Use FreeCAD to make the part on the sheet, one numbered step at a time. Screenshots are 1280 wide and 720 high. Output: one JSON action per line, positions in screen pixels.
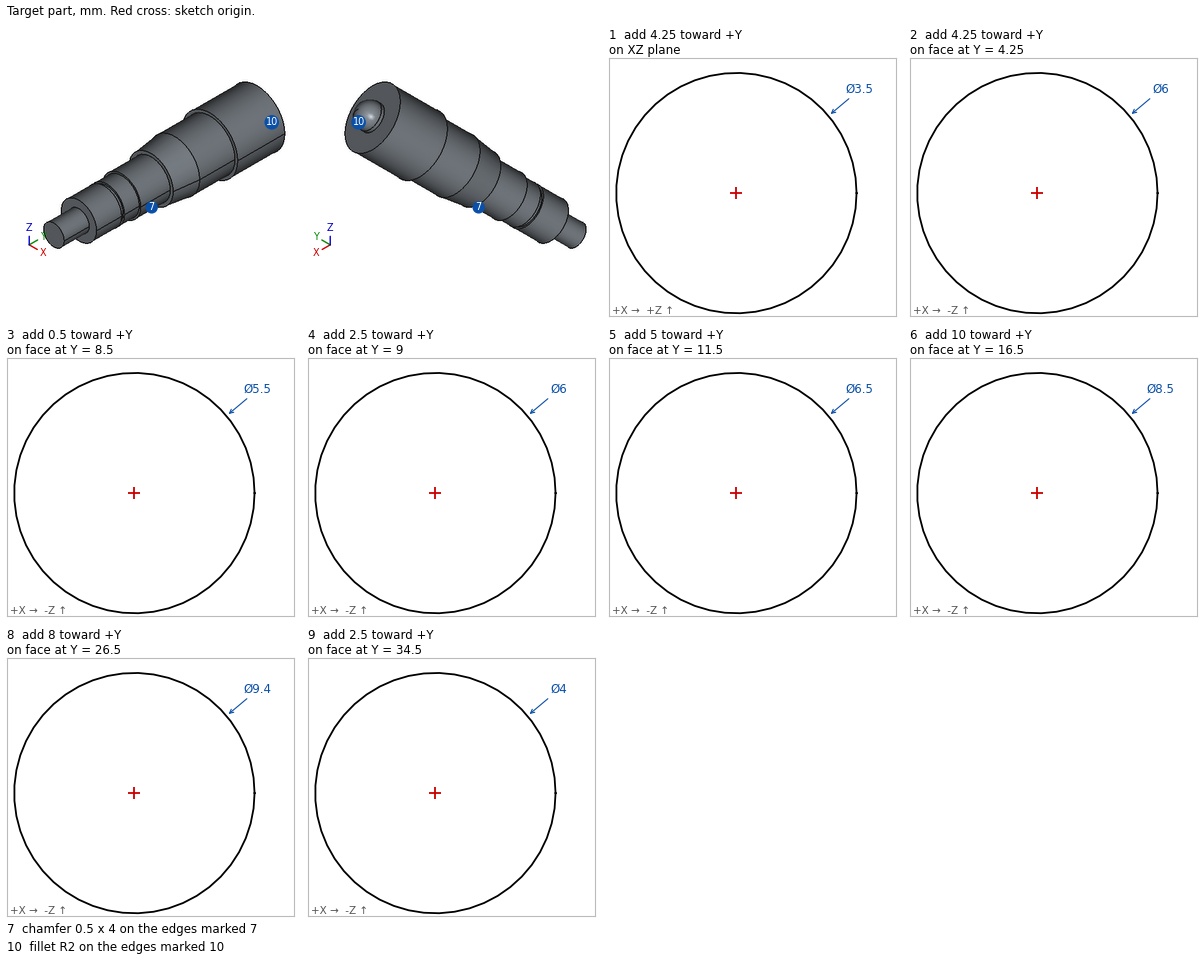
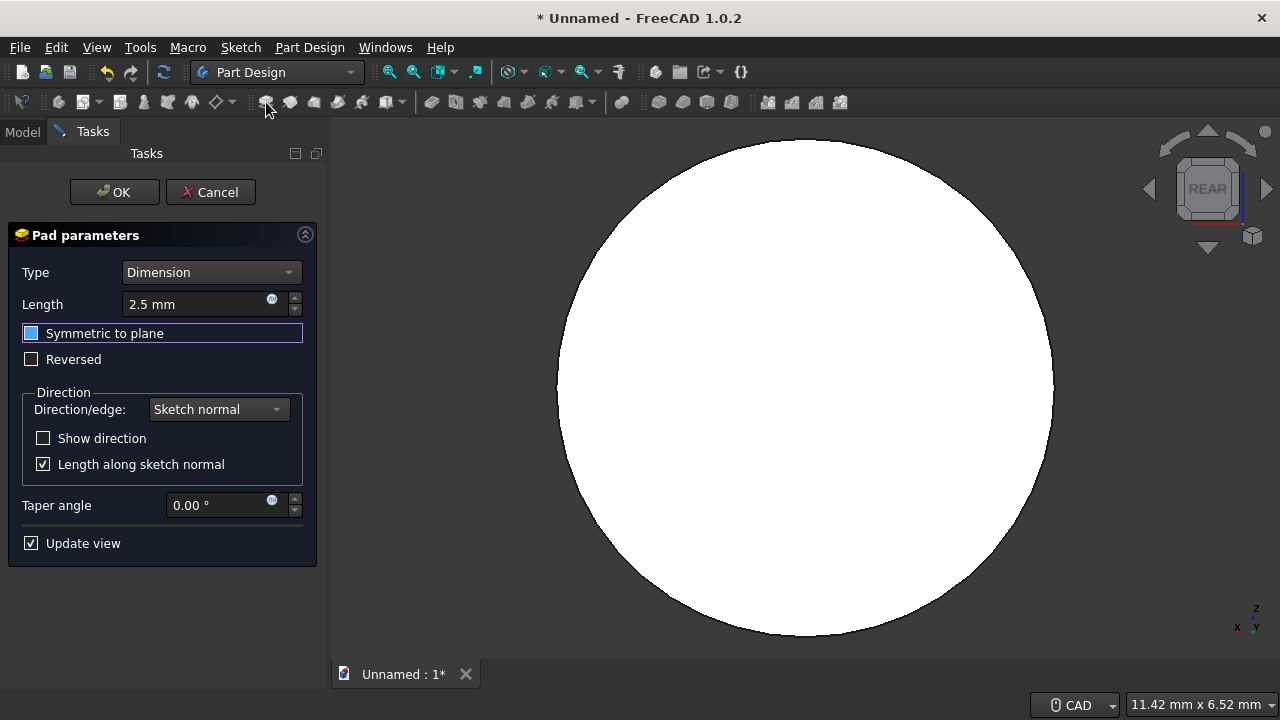
{"action": "left_click", "coordinate": [115, 192]}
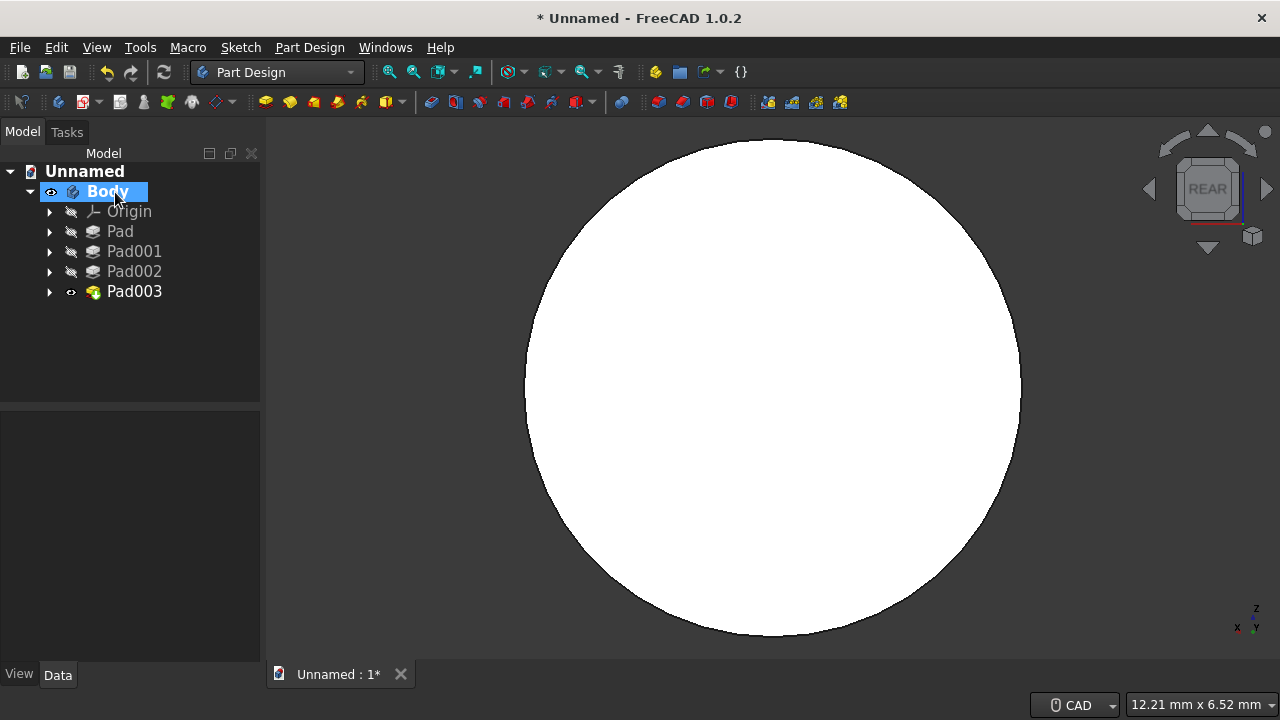
{"action": "left_click", "coordinate": [773, 387]}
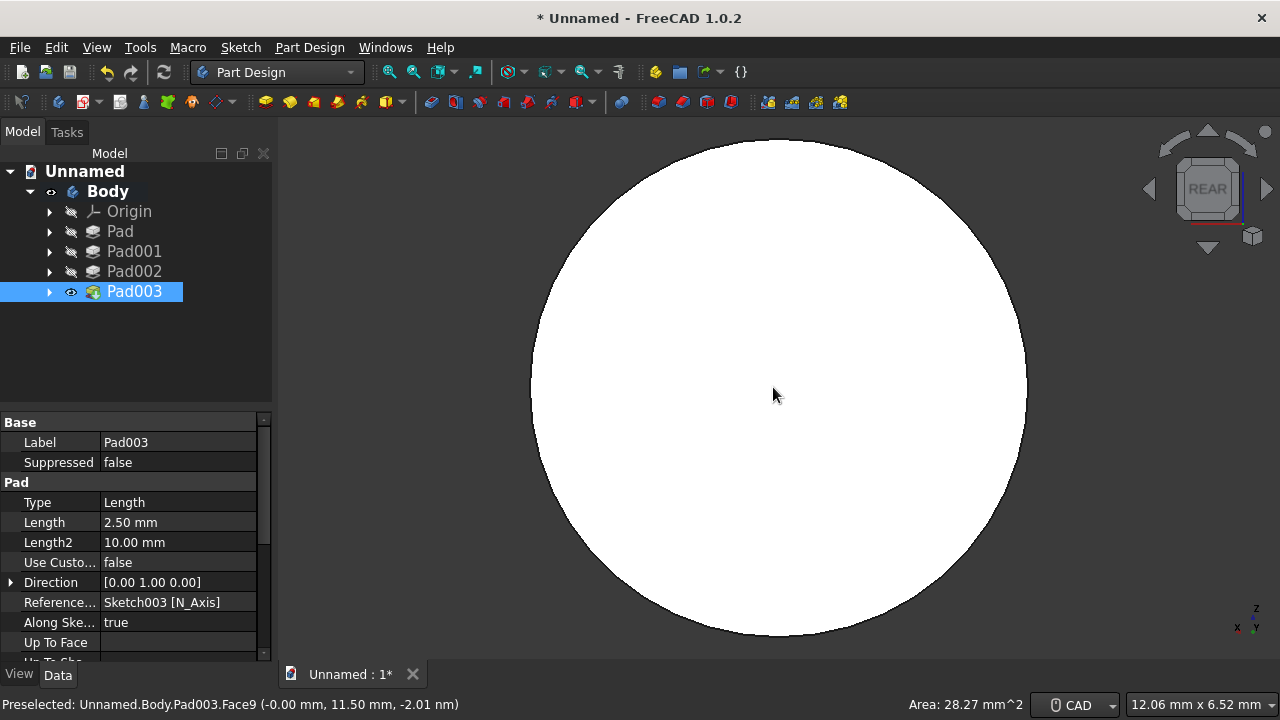
{"action": "left_click", "coordinate": [84, 102]}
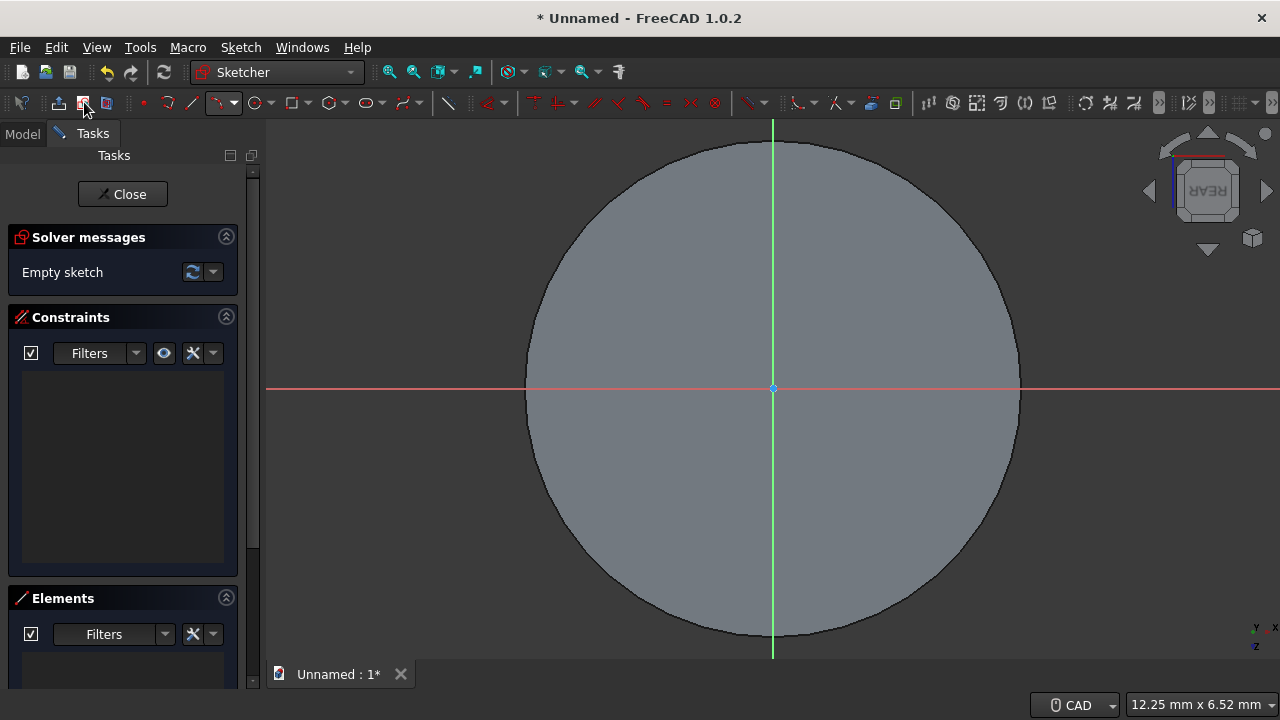
{"action": "scroll", "coordinate": [565, 389], "scroll_direction": "down", "scroll_amount": 2}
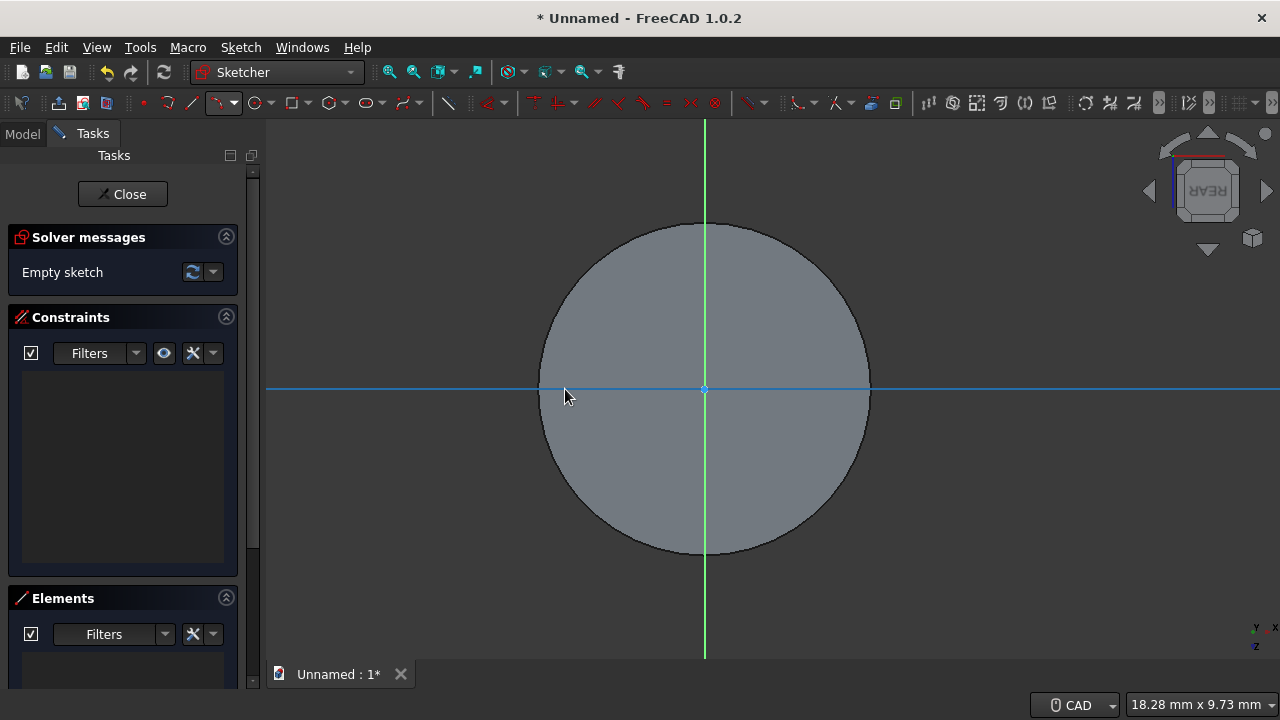
{"action": "left_click", "coordinate": [256, 104]}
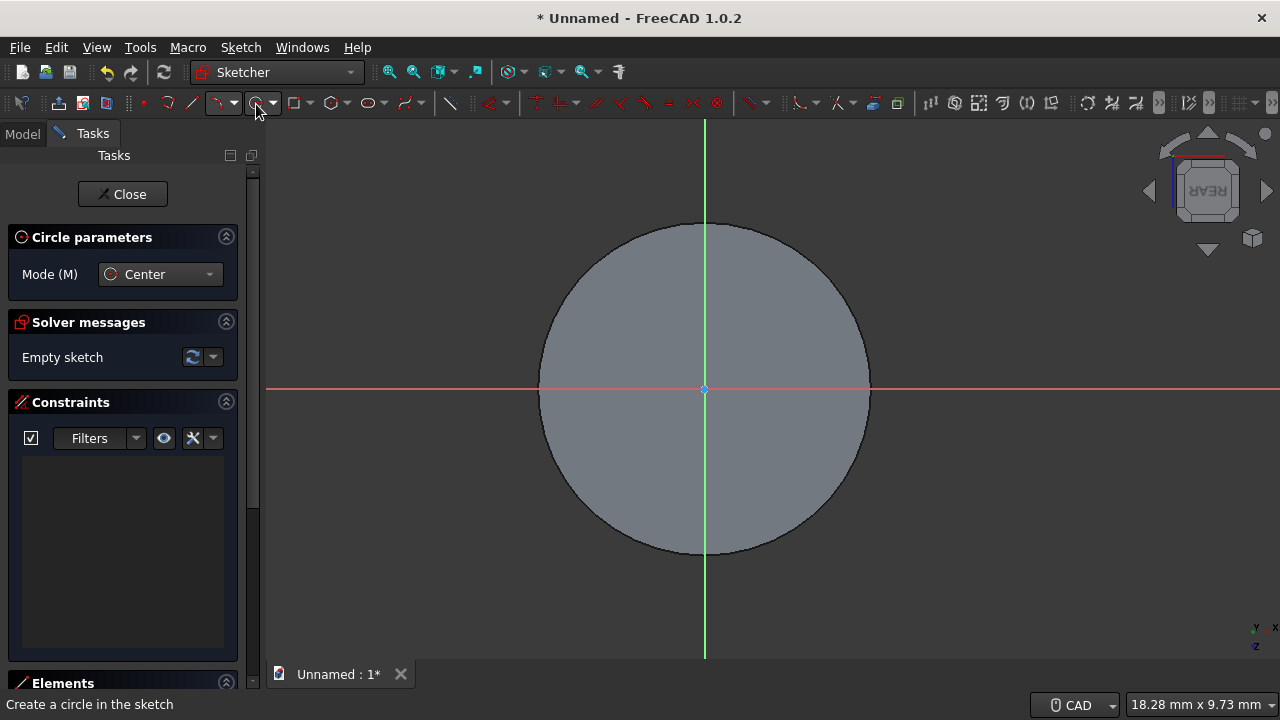
{"action": "left_click", "coordinate": [705, 389]}
{"action": "mouse_move", "coordinate": [832, 262]}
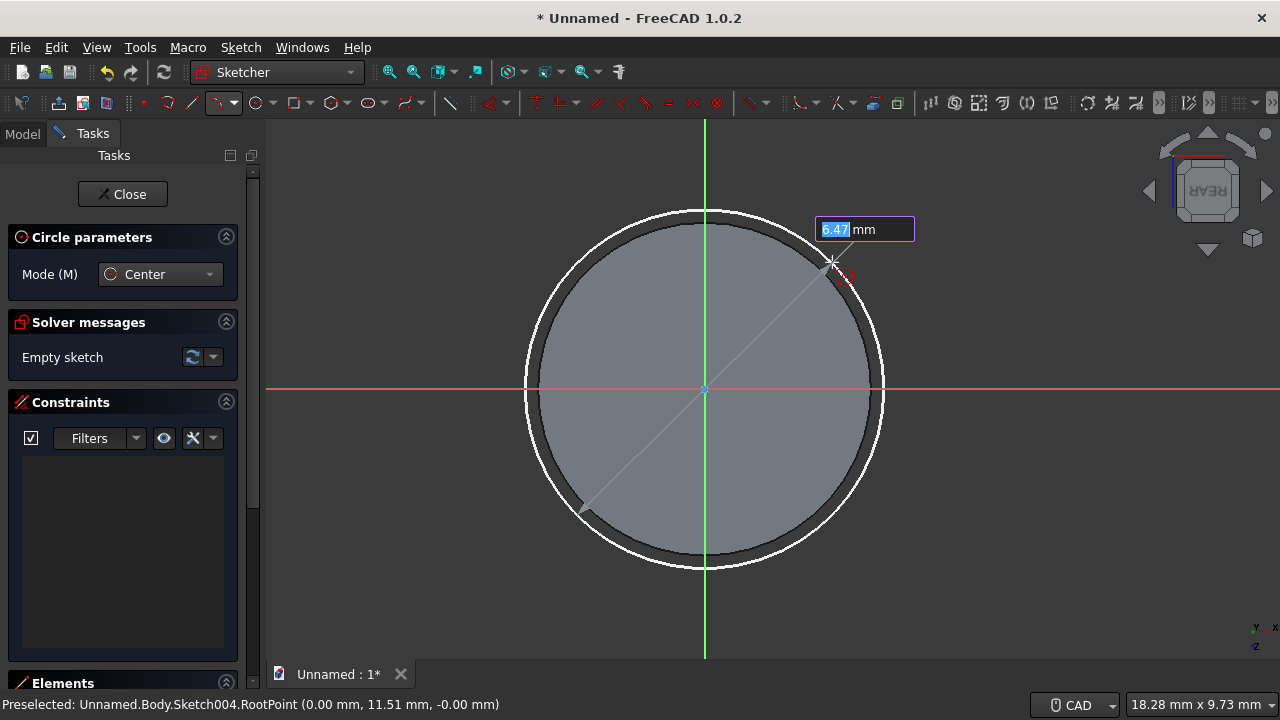
{"action": "type", "text": "6.5"}
{"action": "key", "text": "Return"}
{"action": "key", "text": "Escape"}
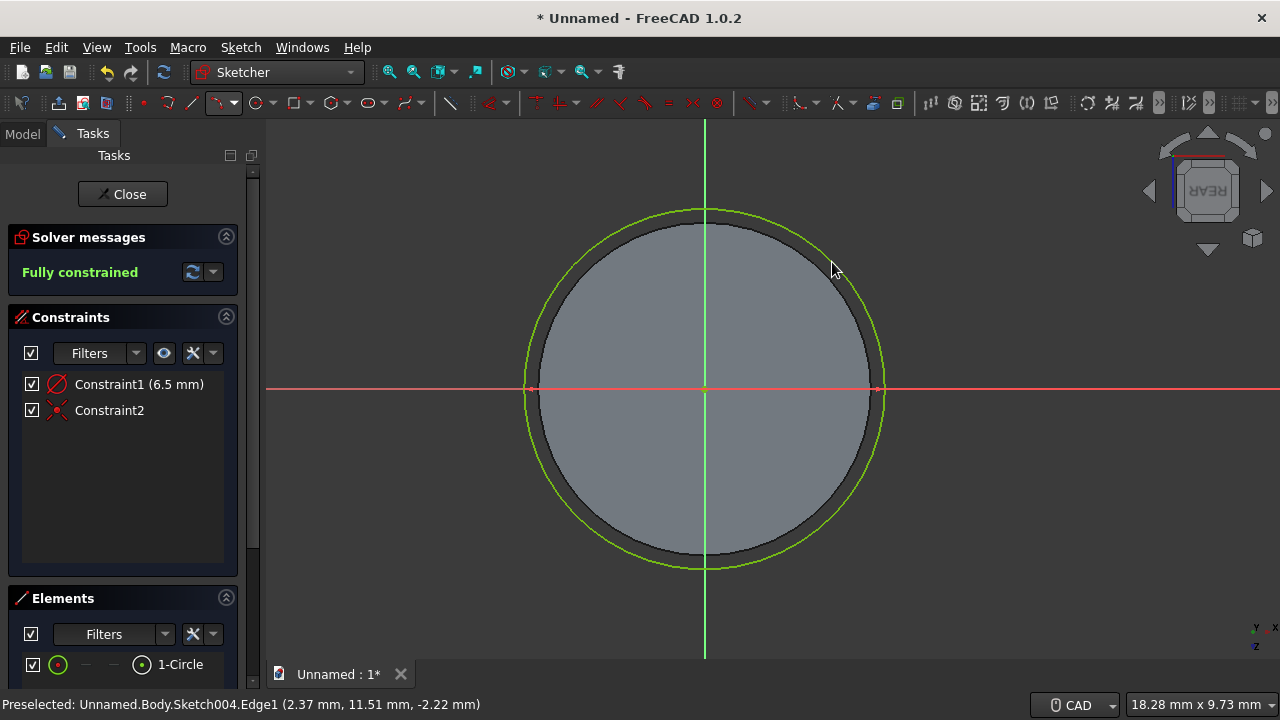
{"action": "left_click", "coordinate": [123, 194]}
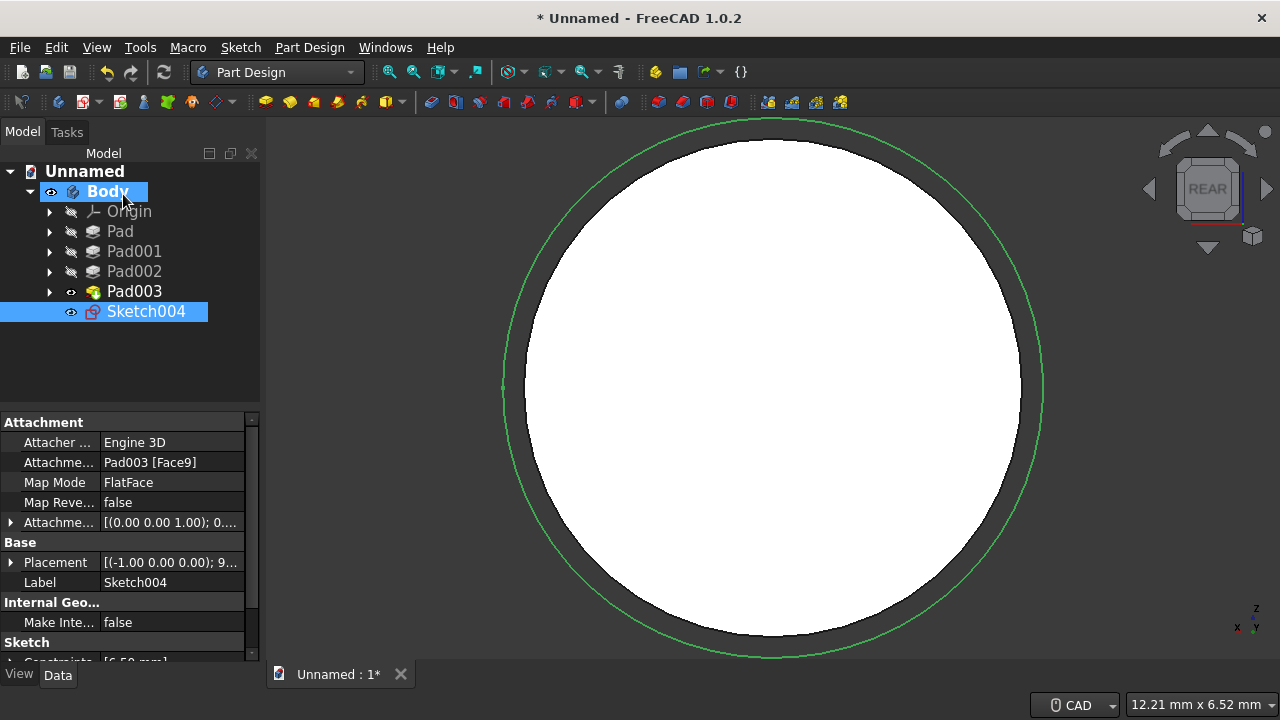
{"action": "left_click", "coordinate": [266, 102]}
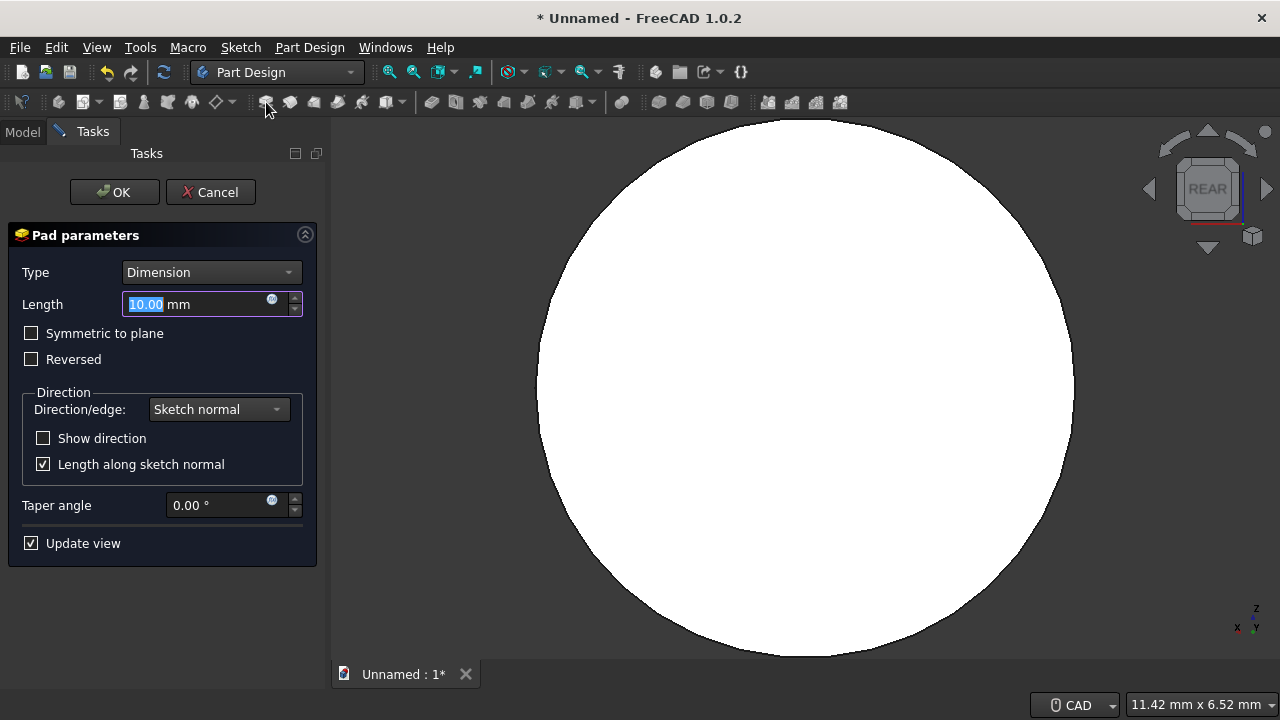
{"action": "type", "text": "5"}
{"action": "key", "text": "Tab"}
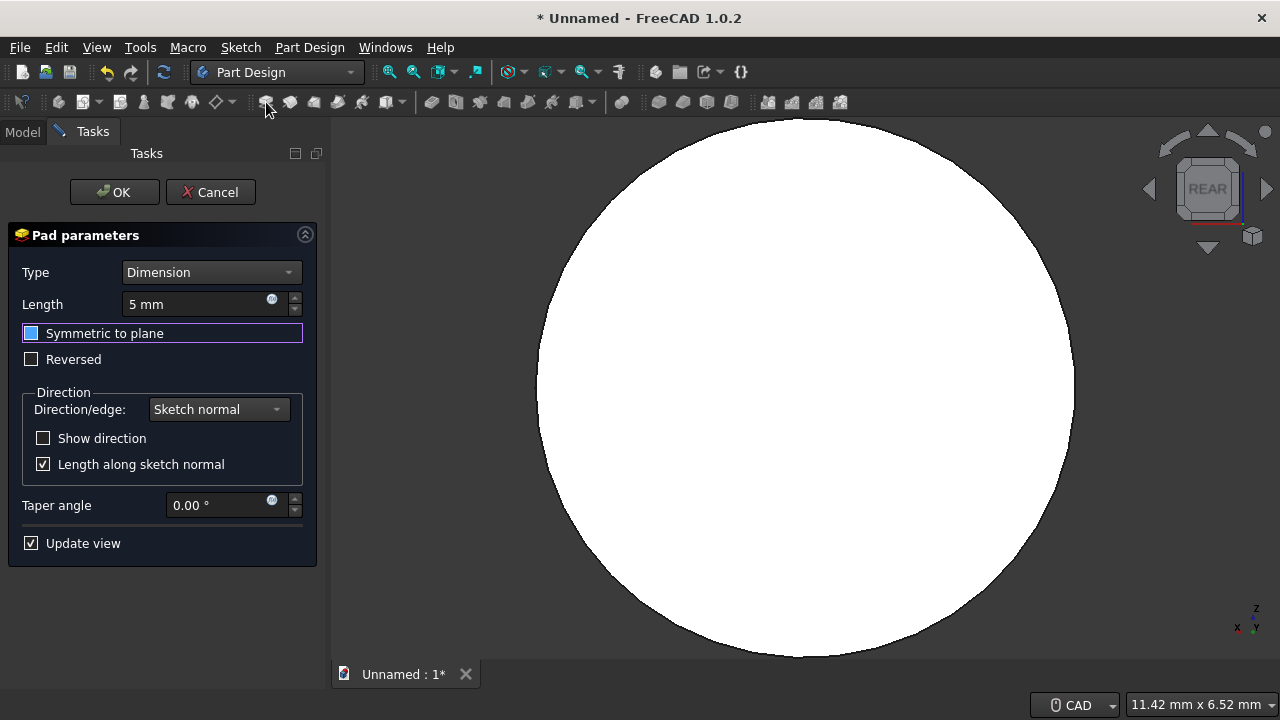
{"action": "left_click", "coordinate": [115, 192]}